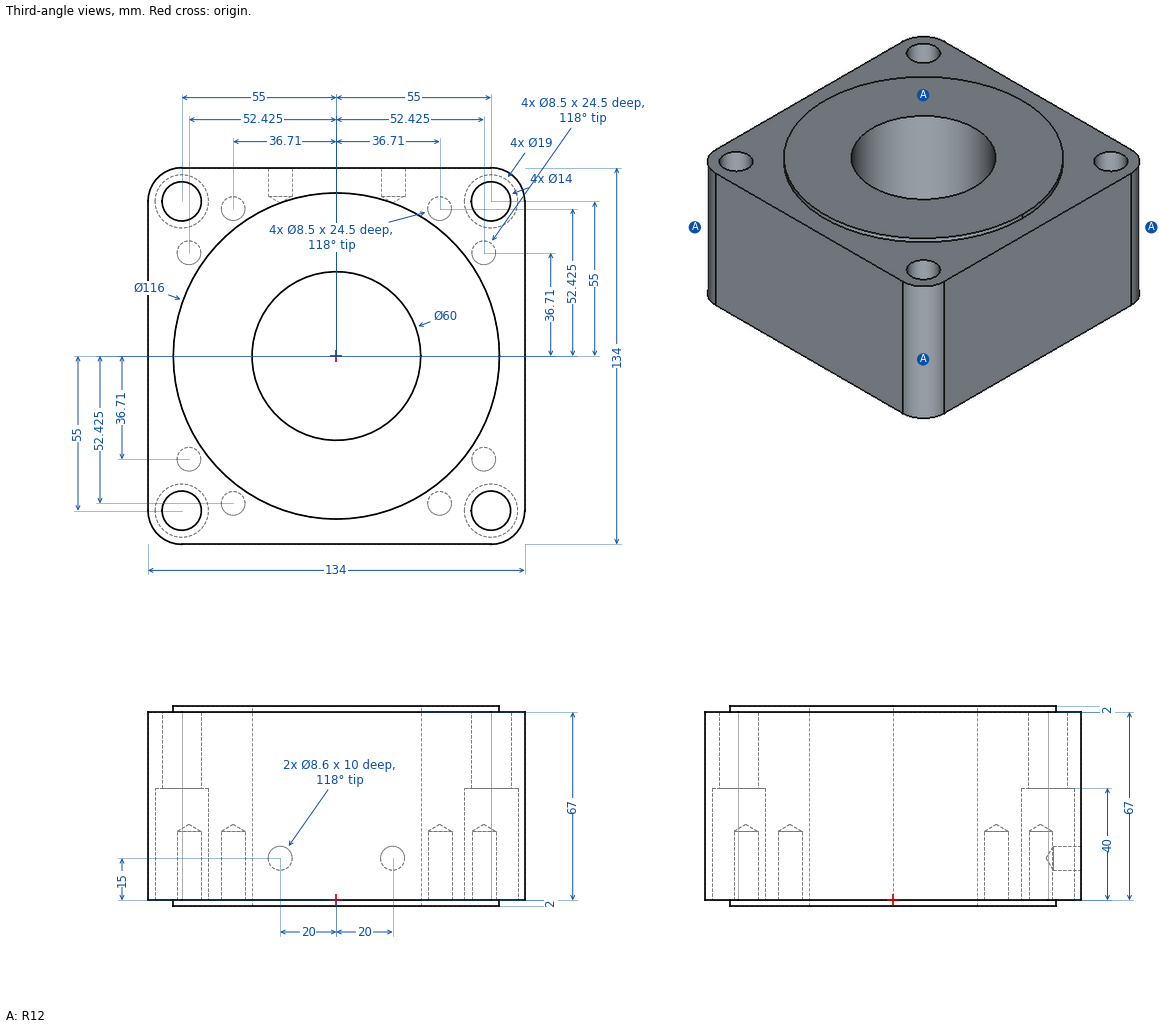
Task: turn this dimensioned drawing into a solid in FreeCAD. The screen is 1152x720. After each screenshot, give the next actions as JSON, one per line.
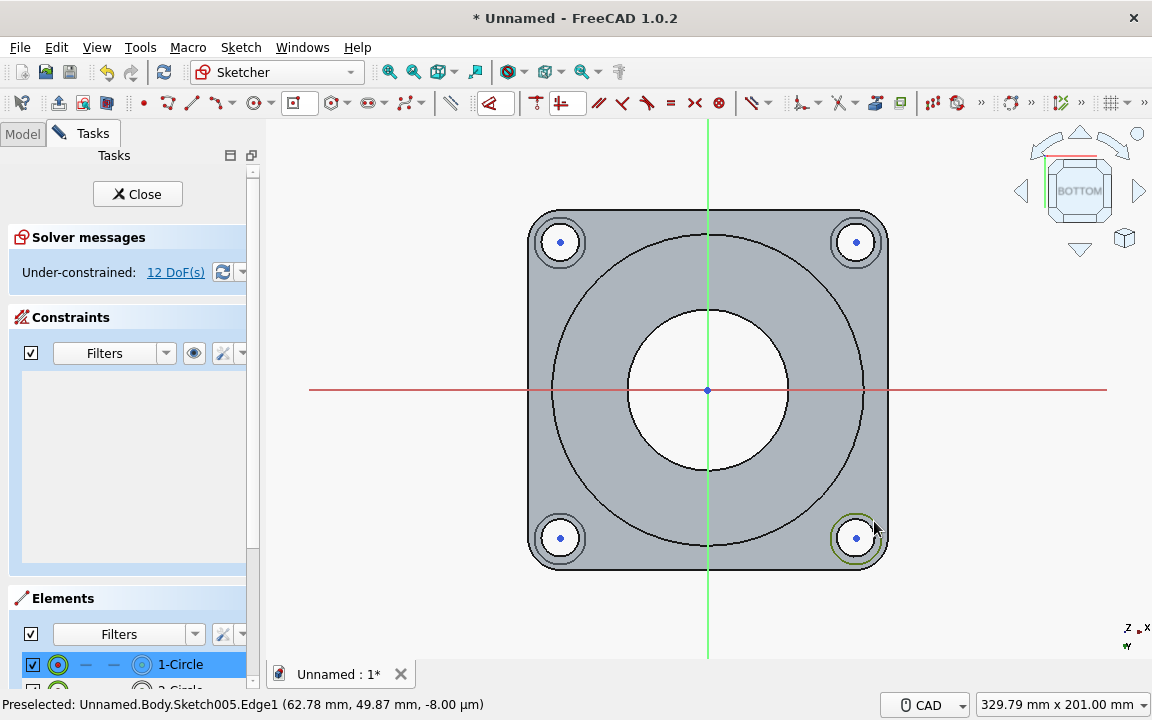
{"action": "left_click", "coordinate": [578, 521]}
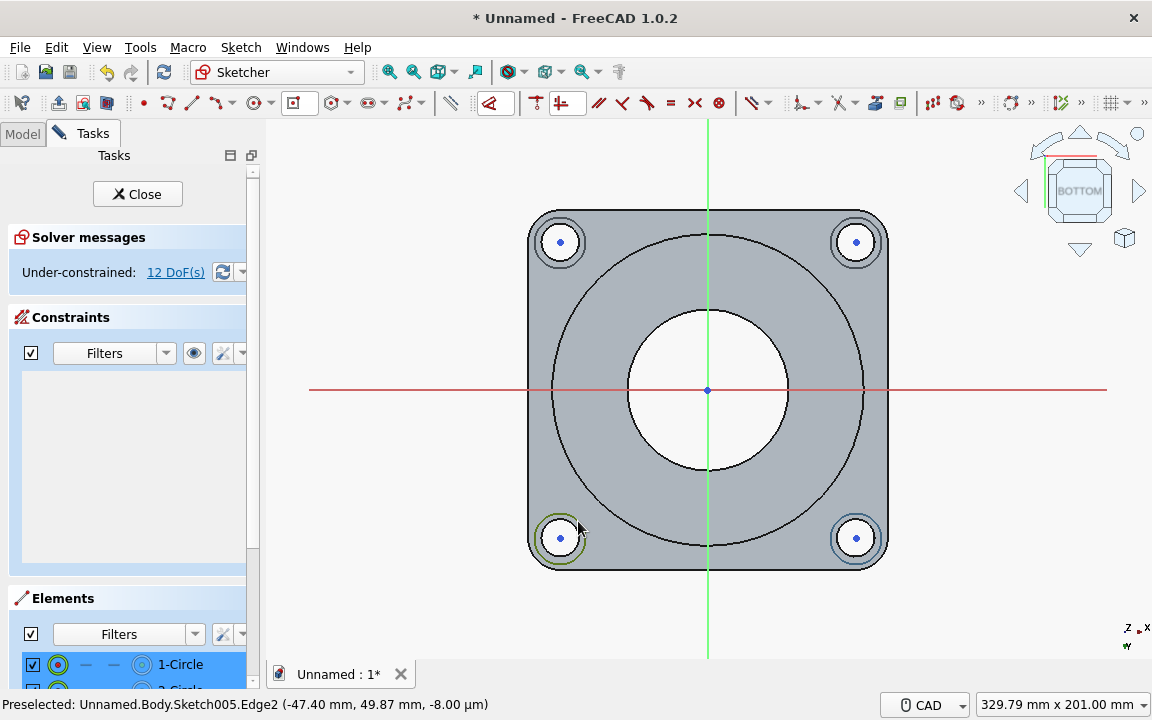
{"action": "left_click", "coordinate": [578, 225]}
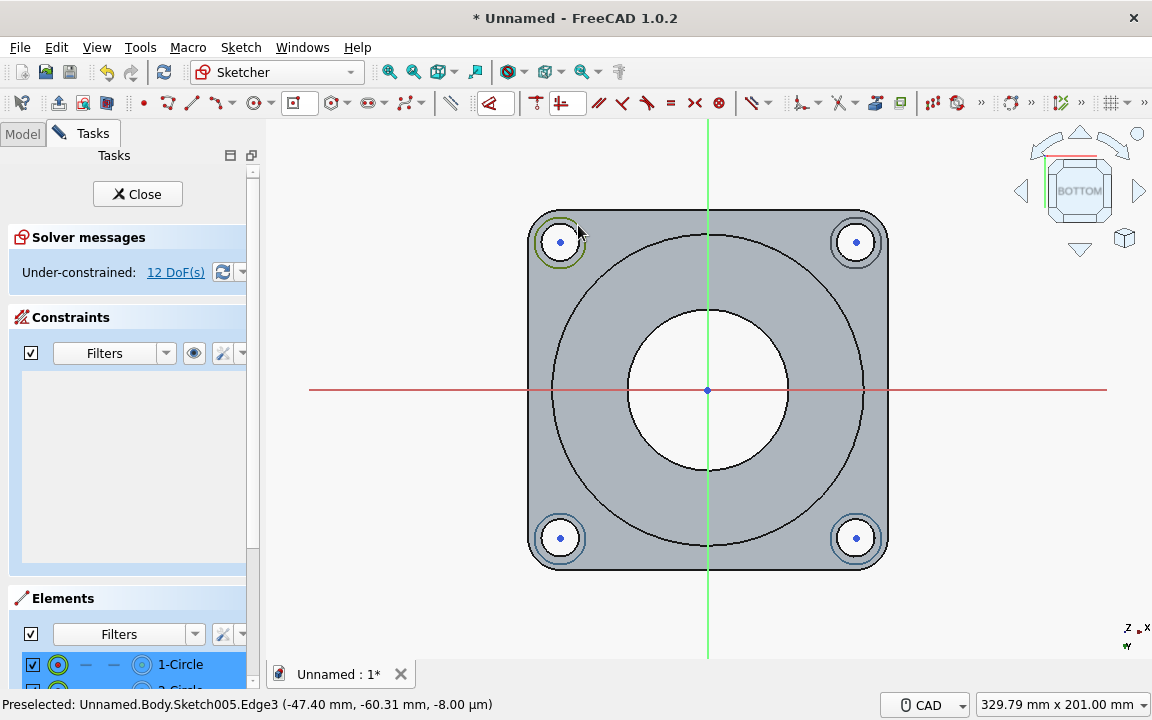
{"action": "left_click", "coordinate": [874, 225]}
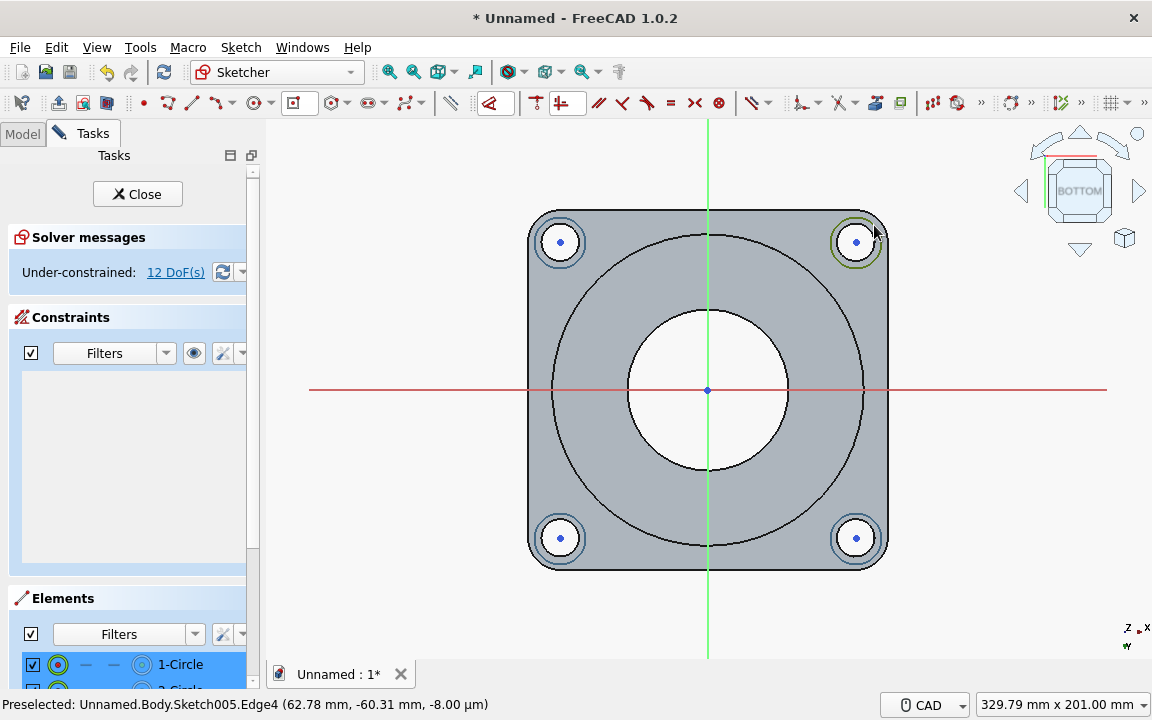
{"action": "left_click", "coordinate": [672, 104]}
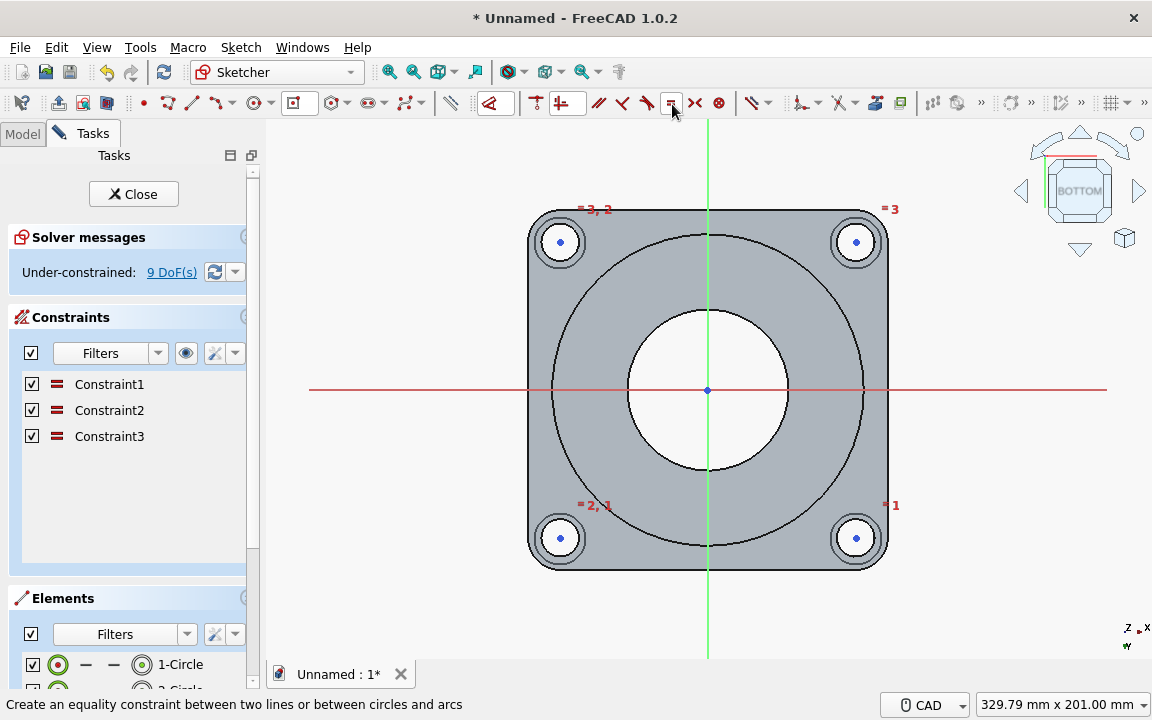
{"action": "left_click", "coordinate": [856, 539]}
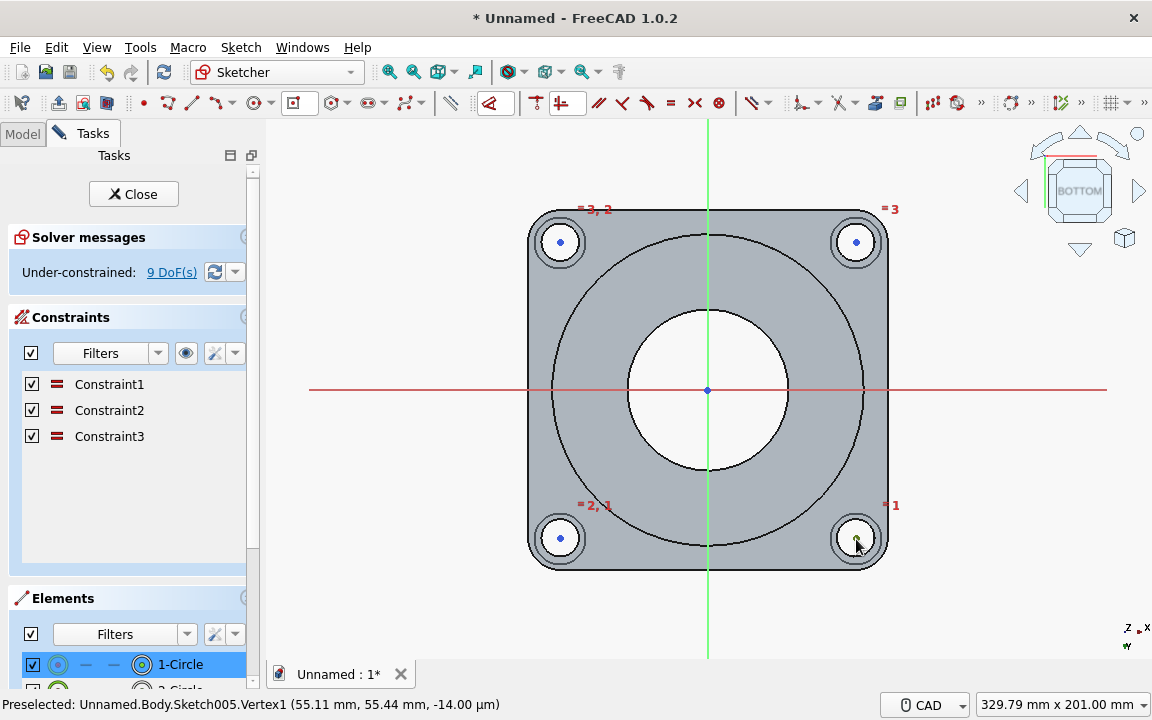
{"action": "left_click", "coordinate": [560, 539]}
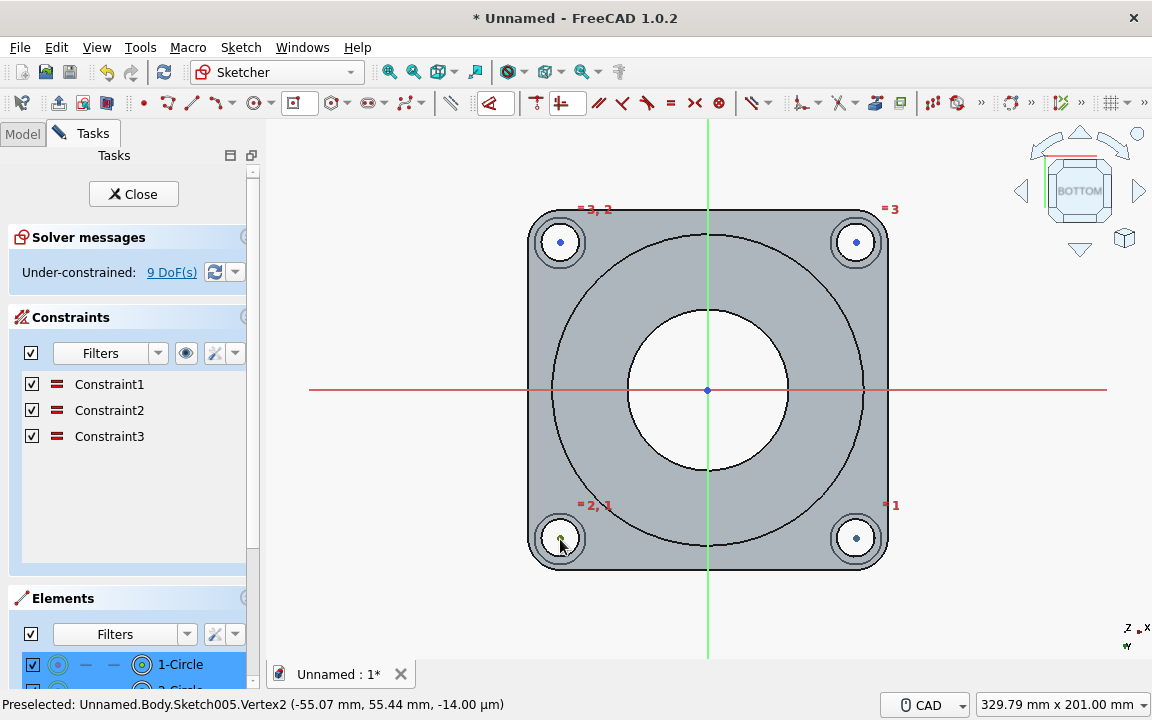
{"action": "key", "text": "h"}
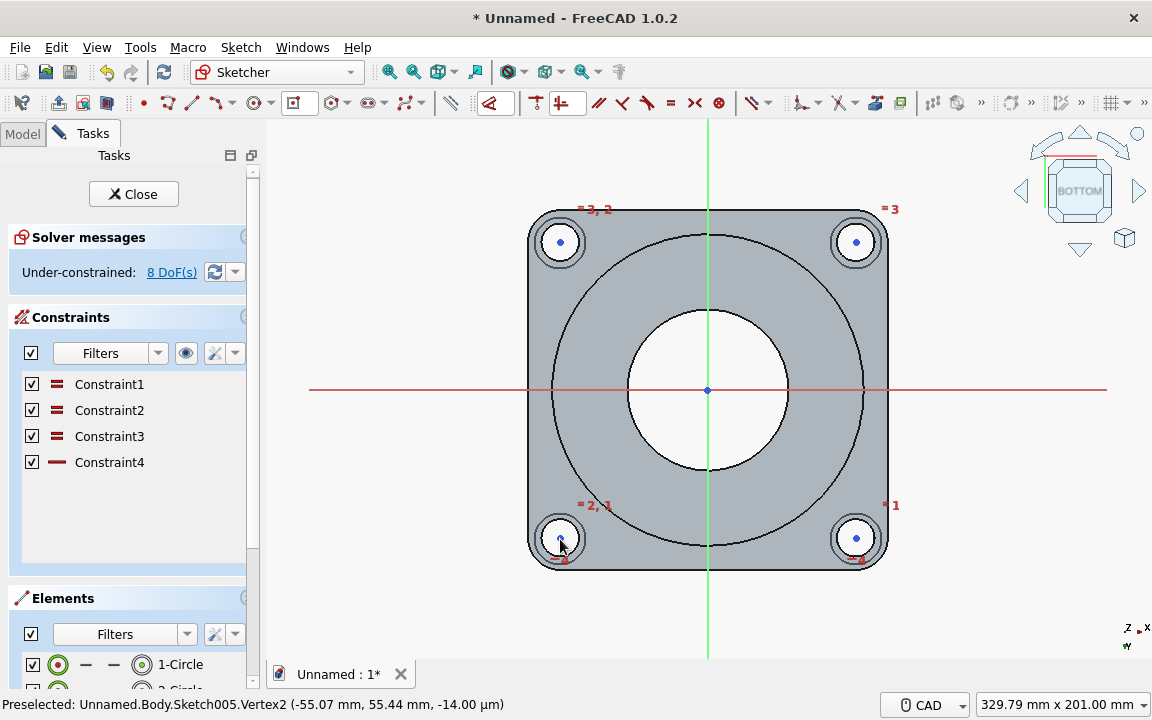
{"action": "left_click", "coordinate": [560, 539]}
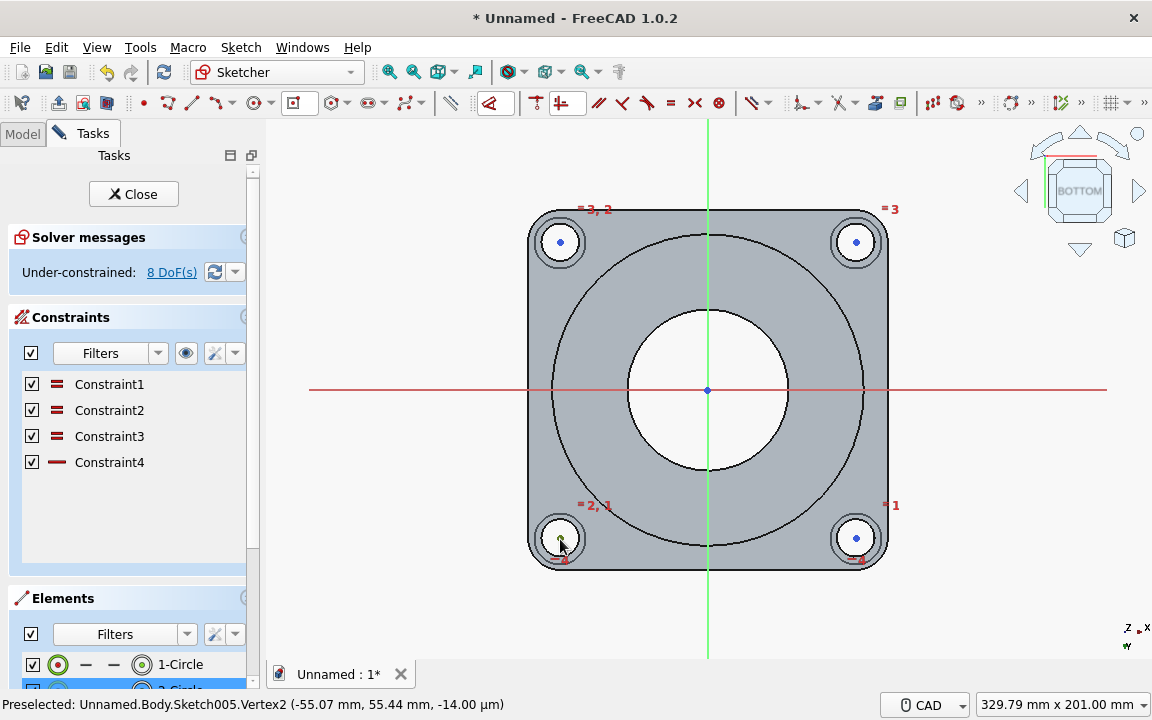
{"action": "left_click", "coordinate": [560, 243]}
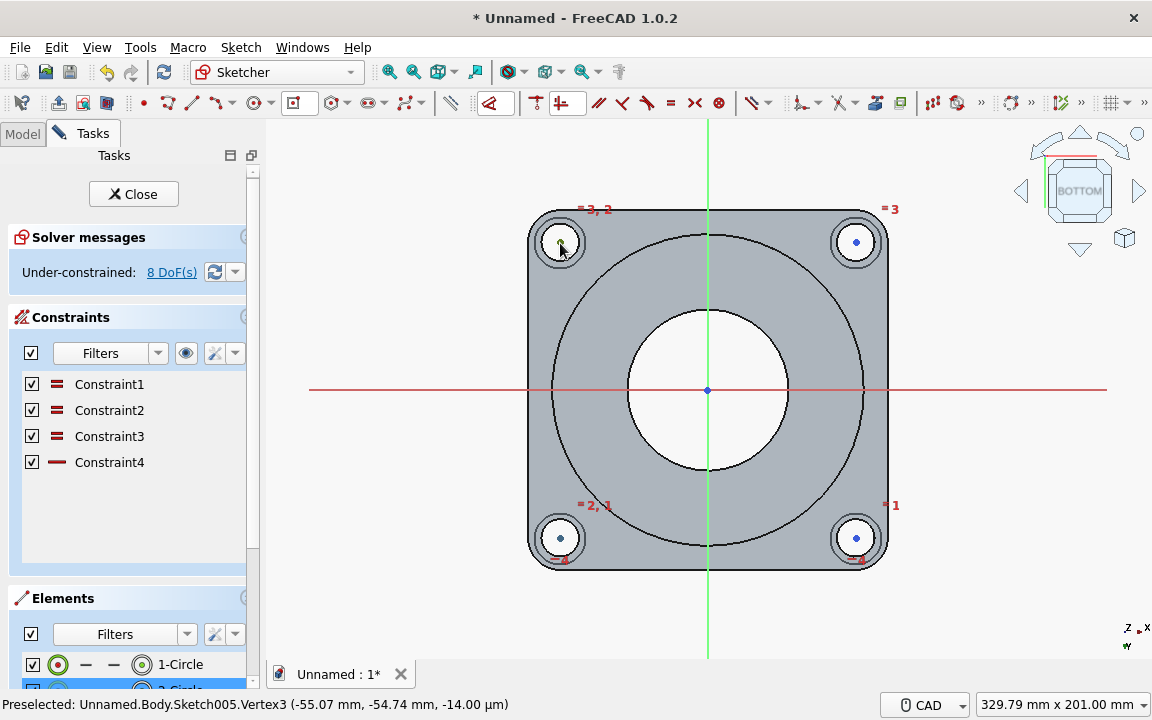
{"action": "left_click", "coordinate": [580, 104]}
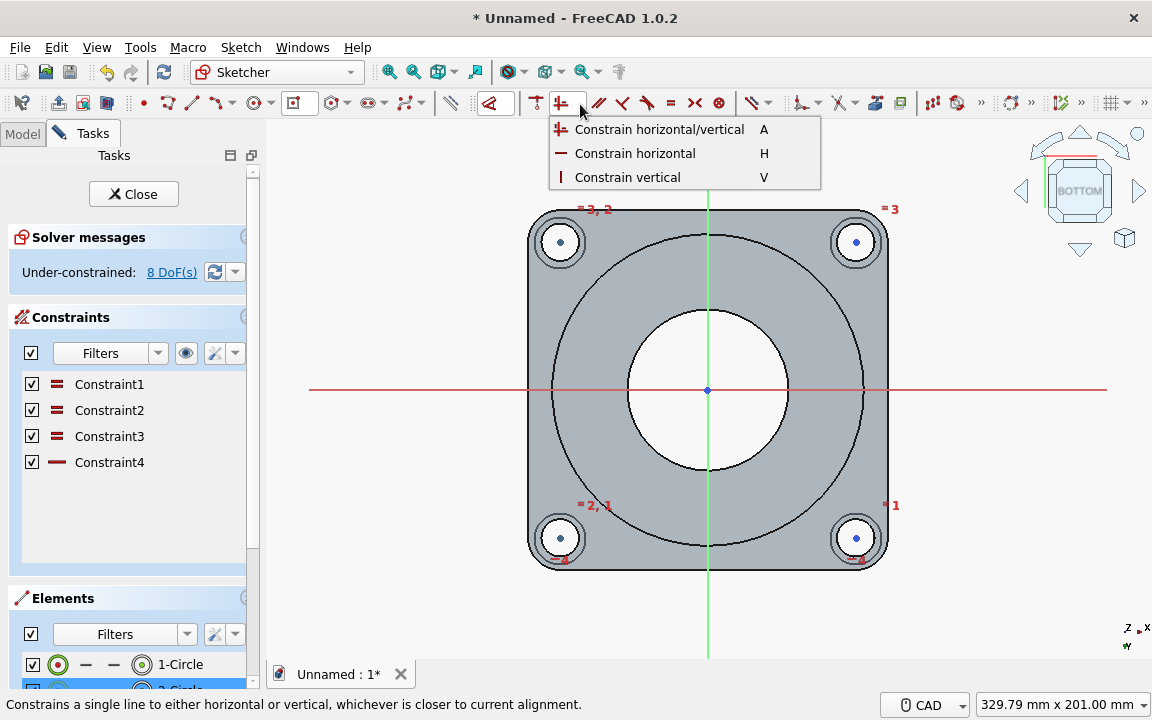
{"action": "left_click", "coordinate": [685, 177]}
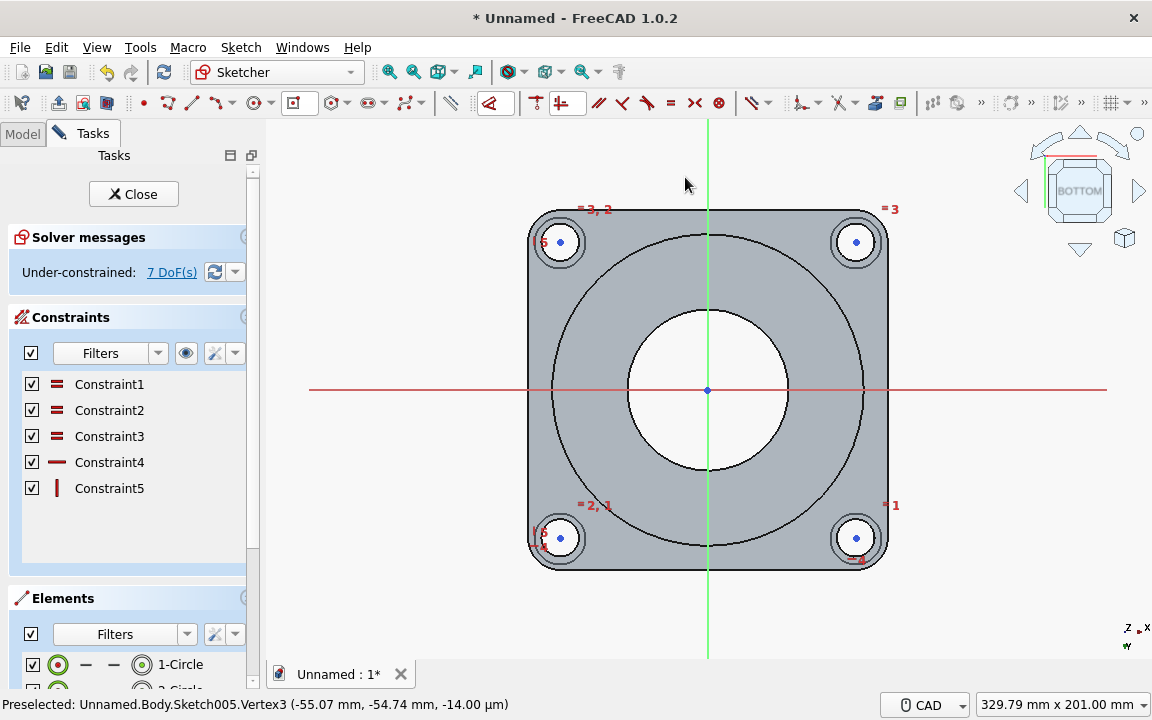
{"action": "left_click", "coordinate": [856, 539]}